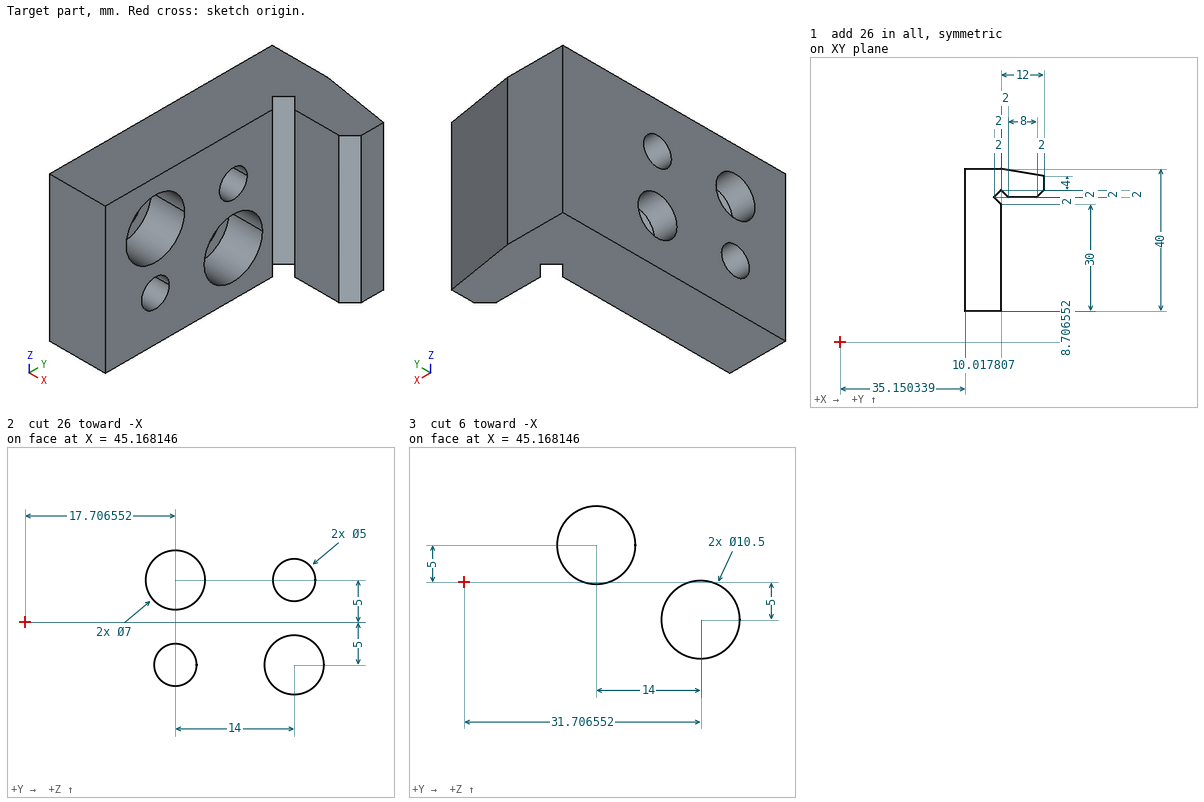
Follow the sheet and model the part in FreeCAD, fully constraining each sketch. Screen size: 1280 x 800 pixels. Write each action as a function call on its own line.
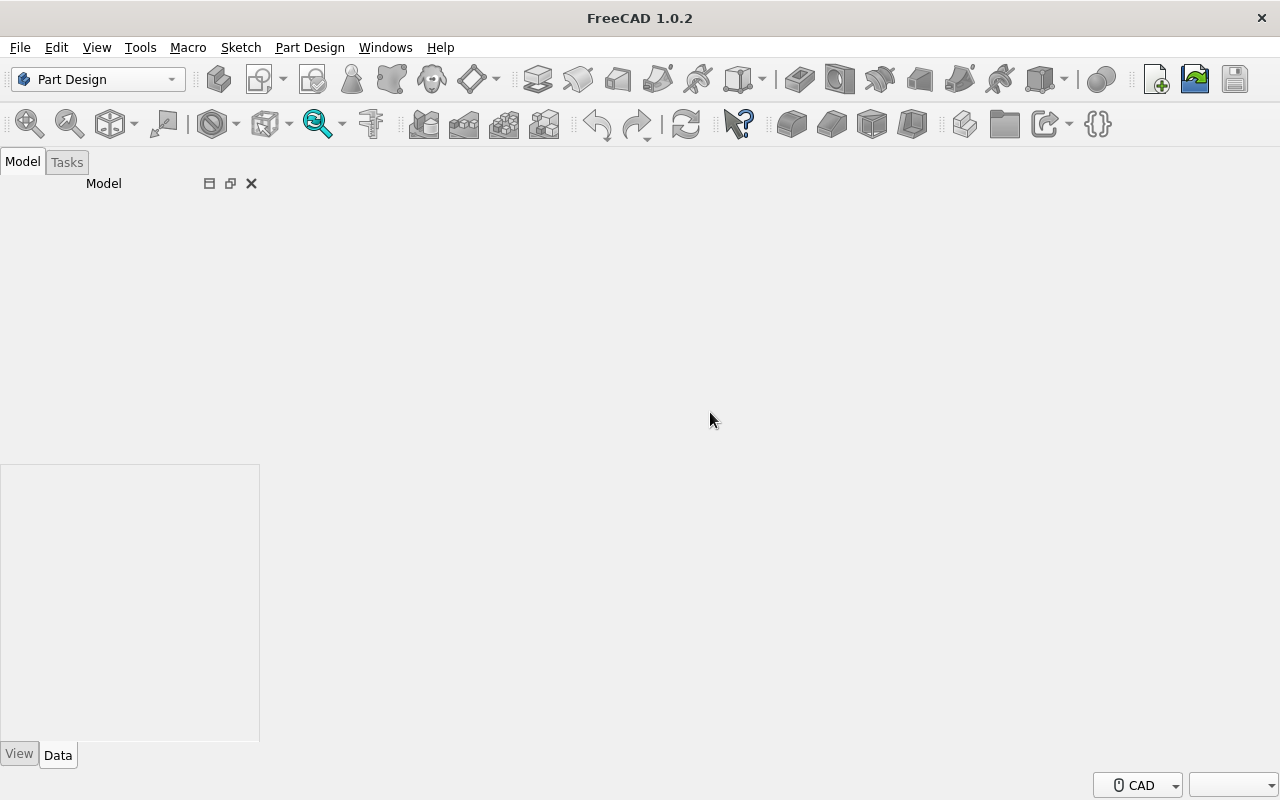
click(1156, 80)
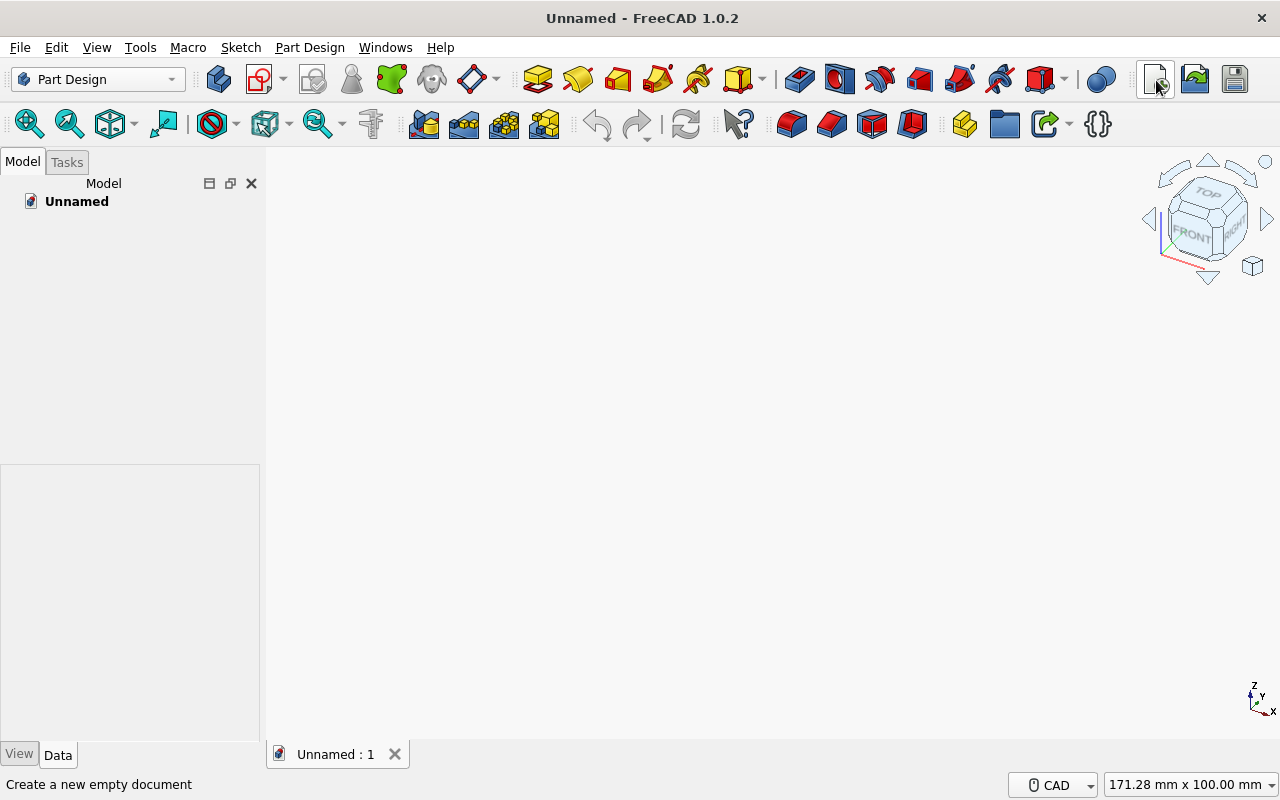
click(260, 80)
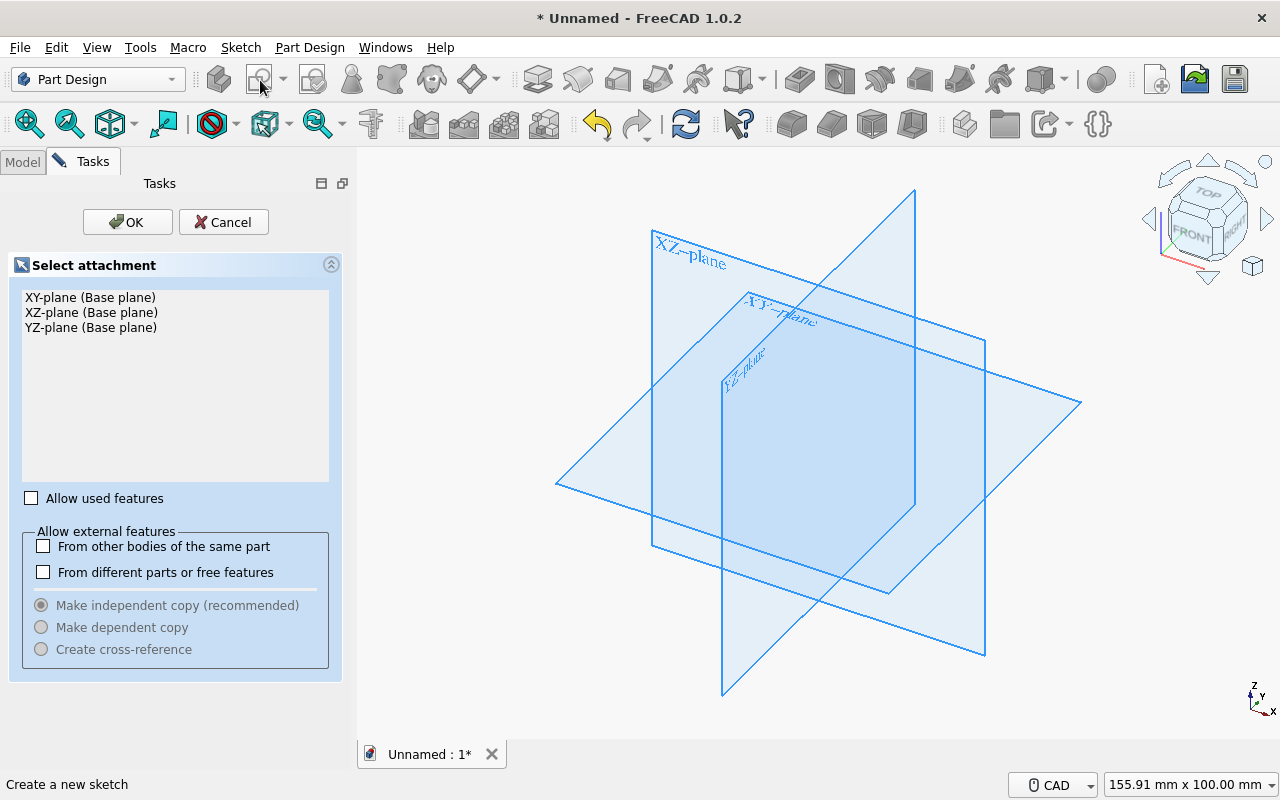
click(82, 298)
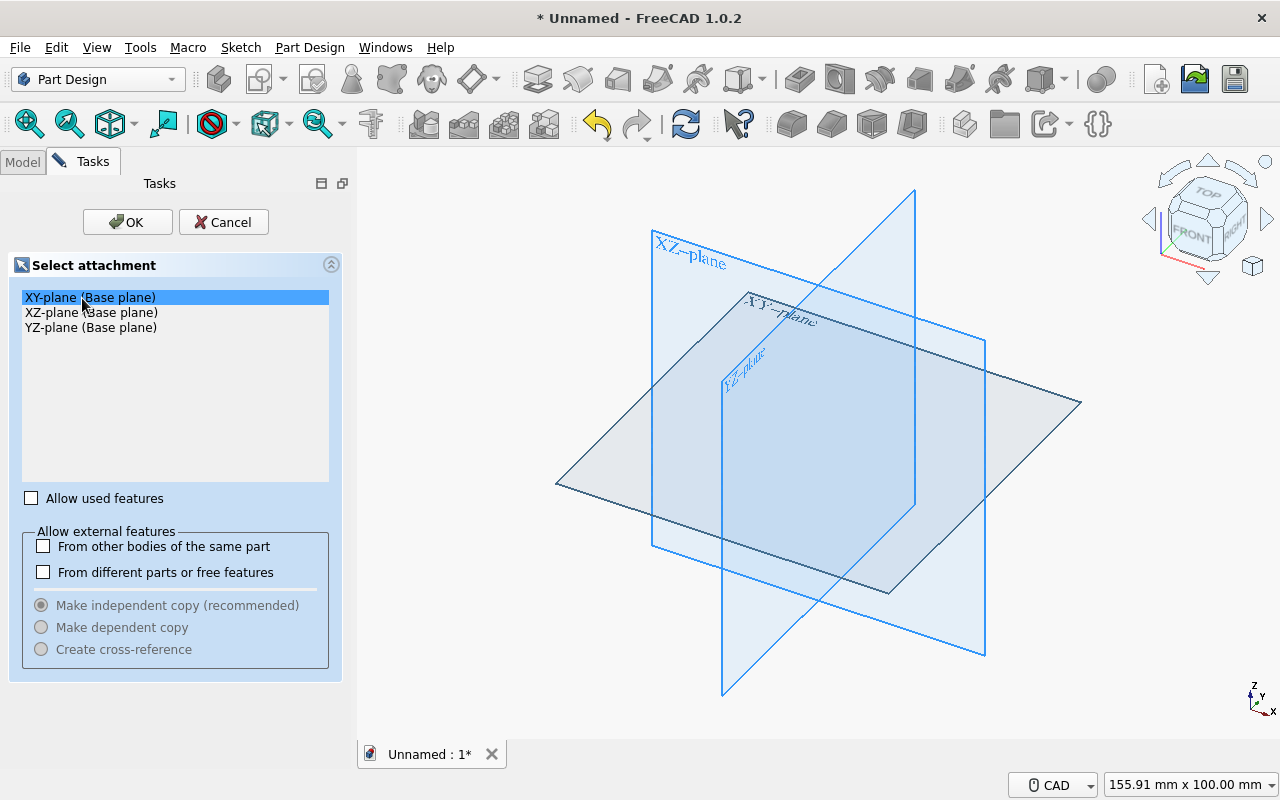
click(128, 222)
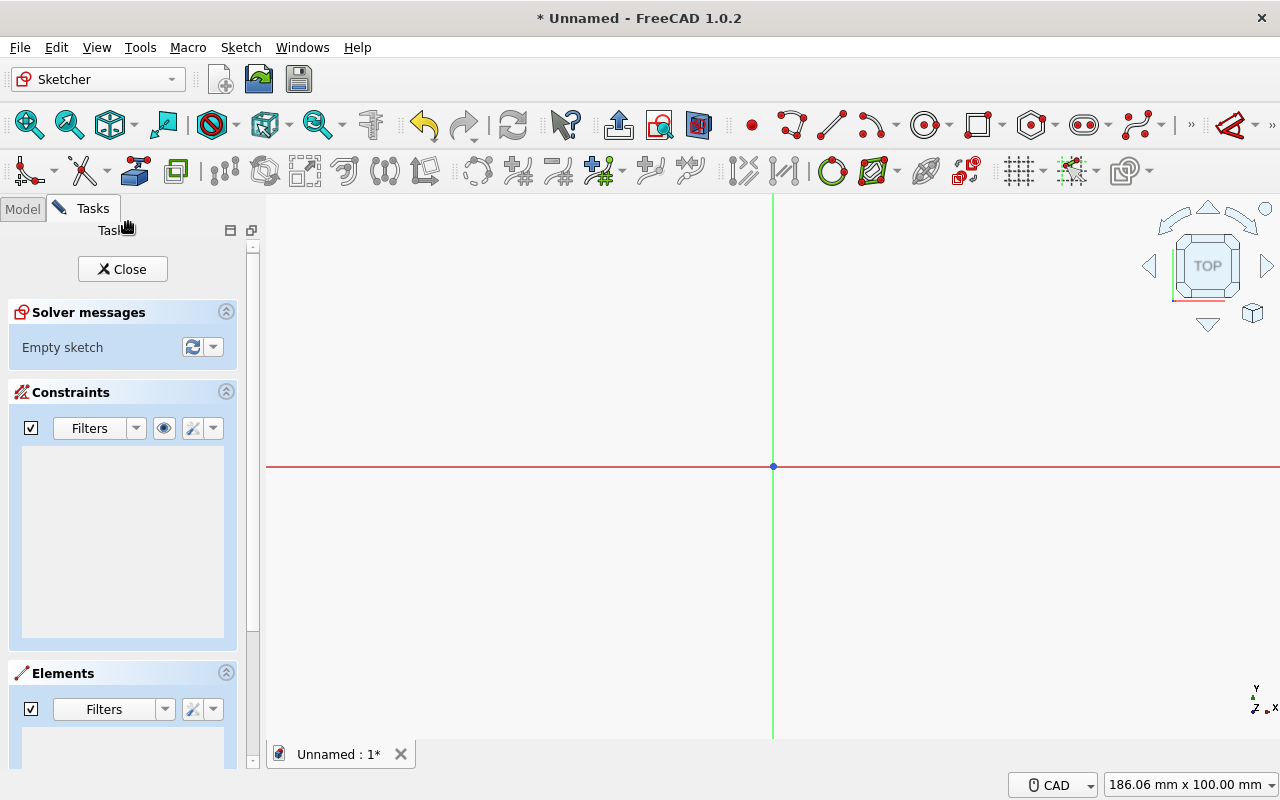
scroll(294, 711, down, 1)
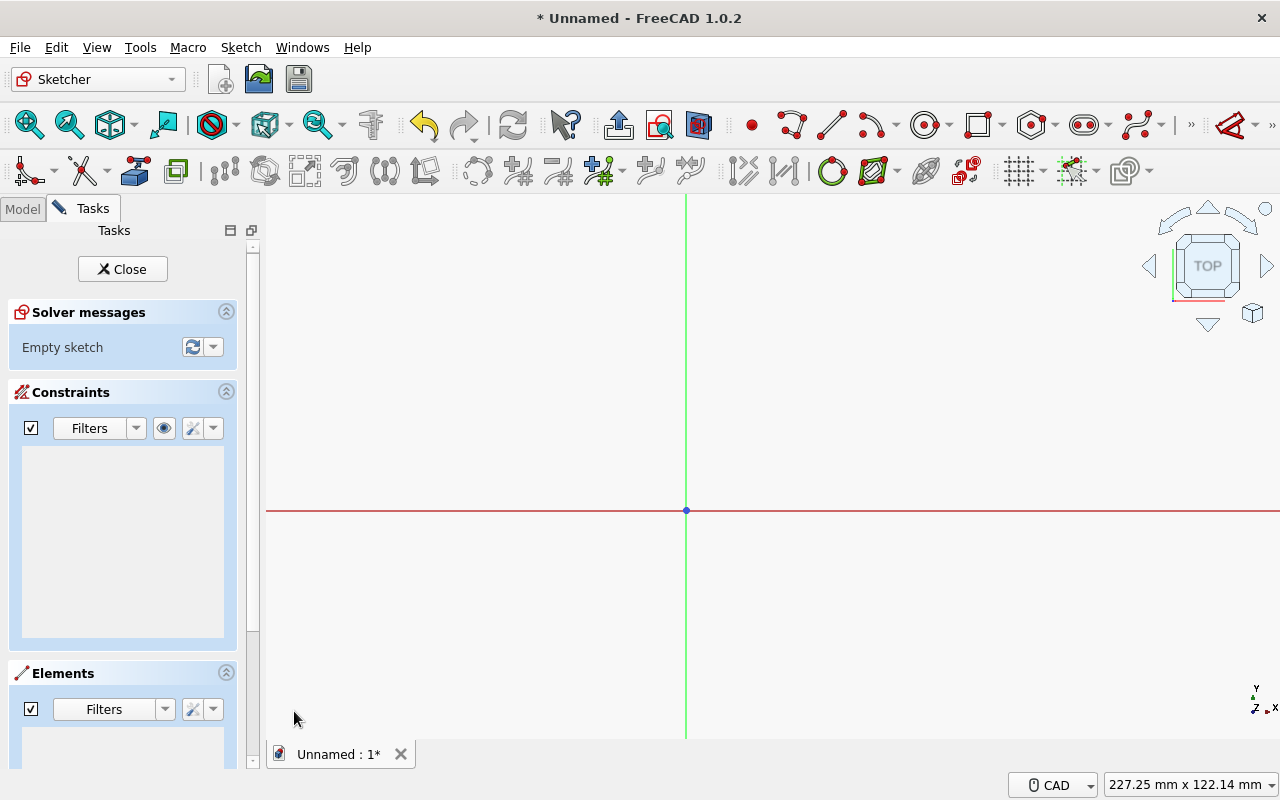
scroll(1036, 272, up, 2)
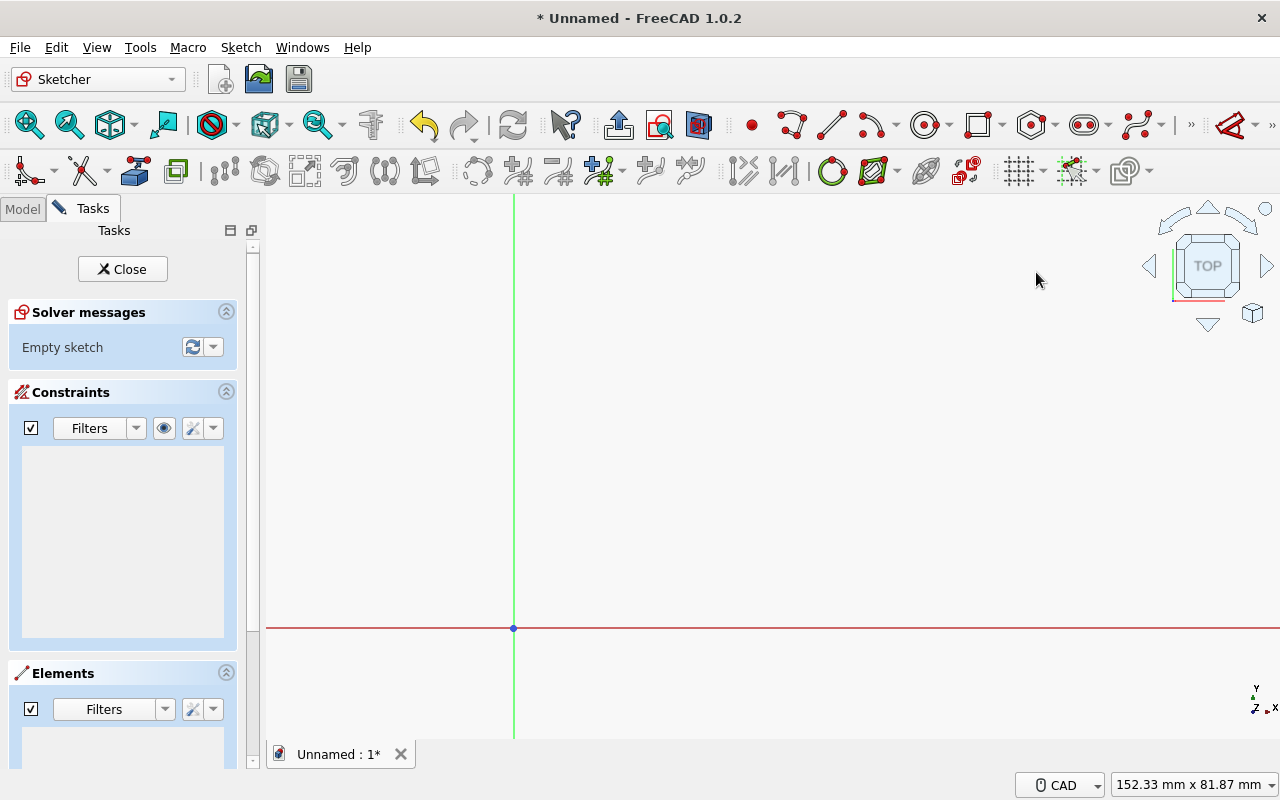
key(g)
key(m)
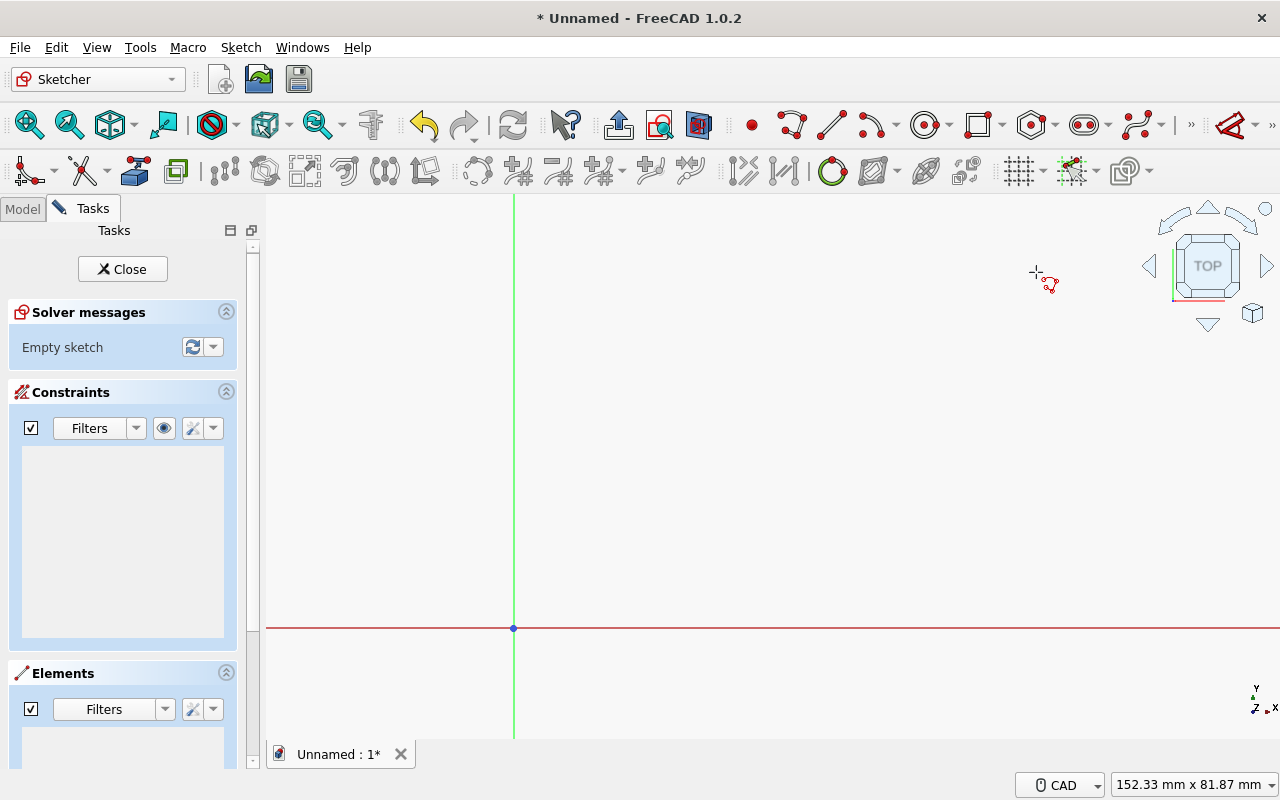
click(748, 571)
click(814, 571)
click(814, 371)
click(801, 357)
click(814, 344)
click(828, 357)
click(881, 357)
click(894, 344)
click(894, 318)
click(814, 304)
click(748, 304)
click(748, 572)
key(Escape)
key(Escape)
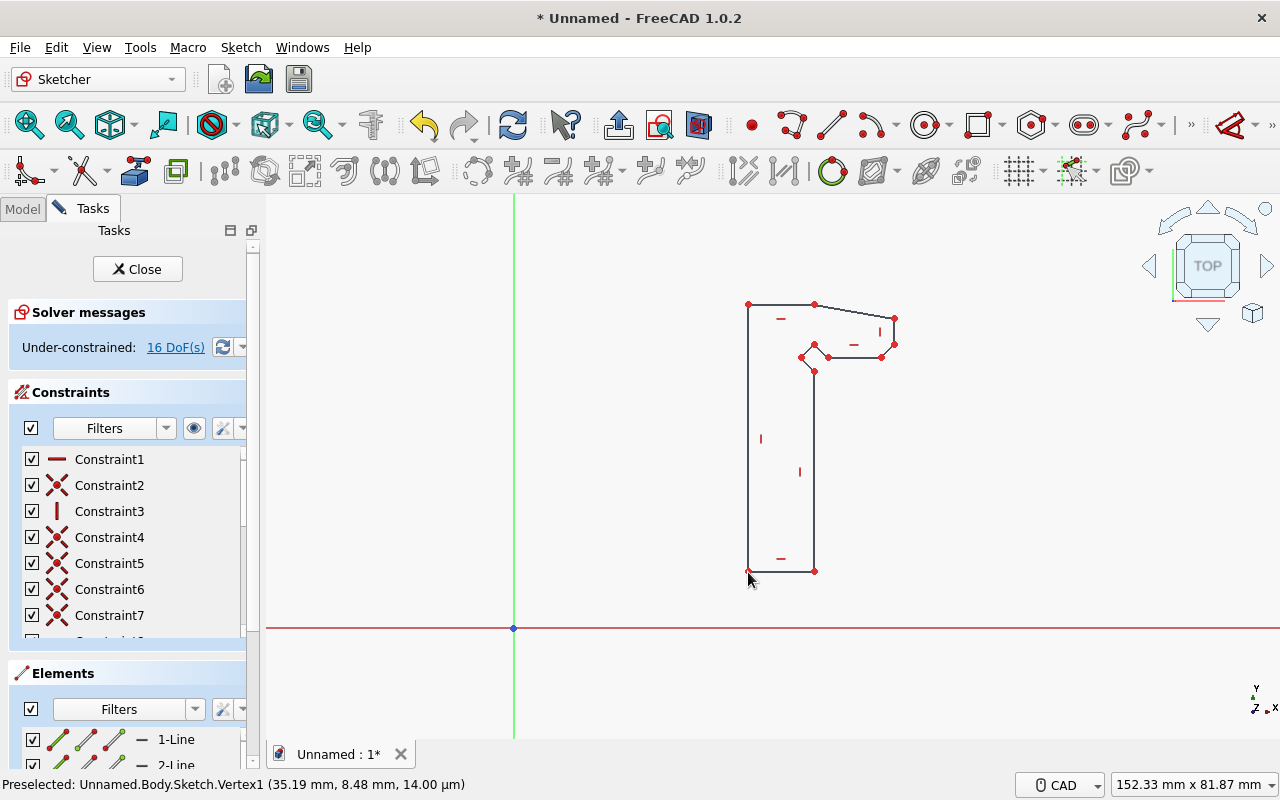
key(d)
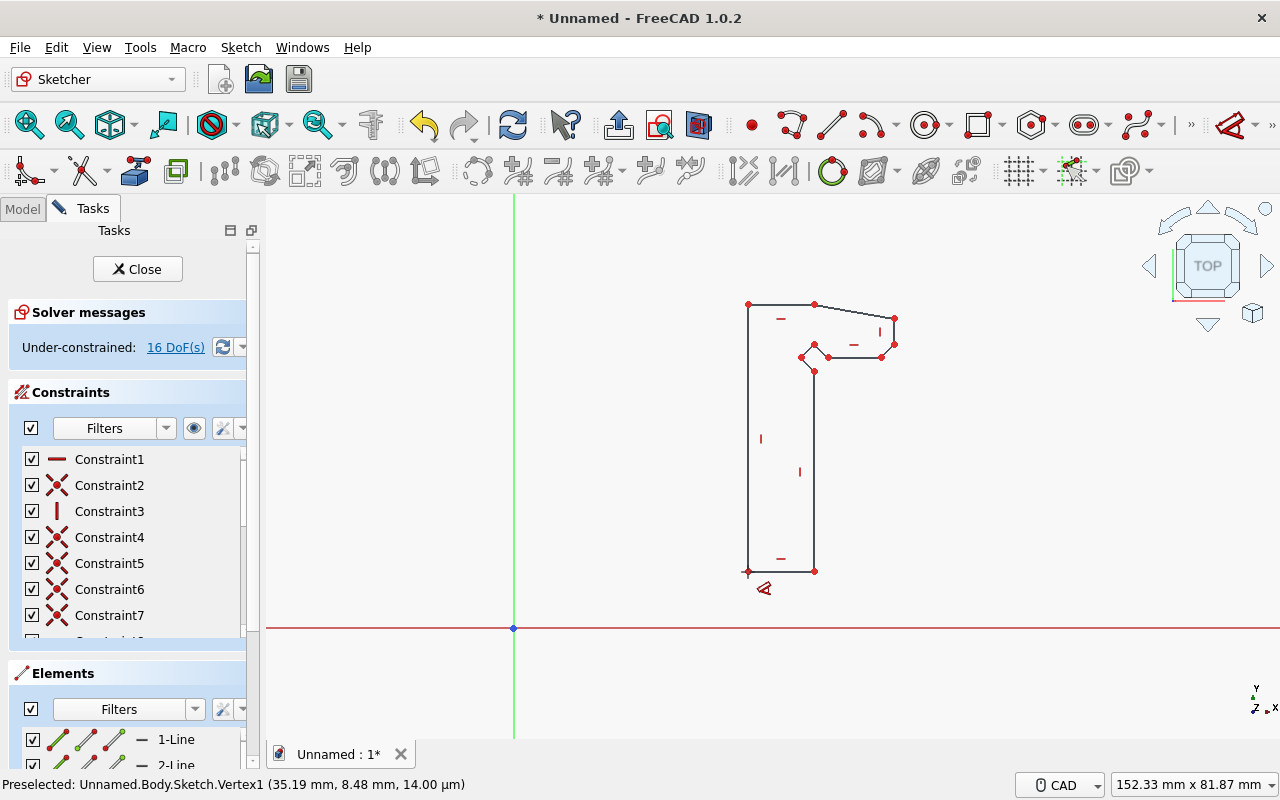
click(844, 358)
click(842, 324)